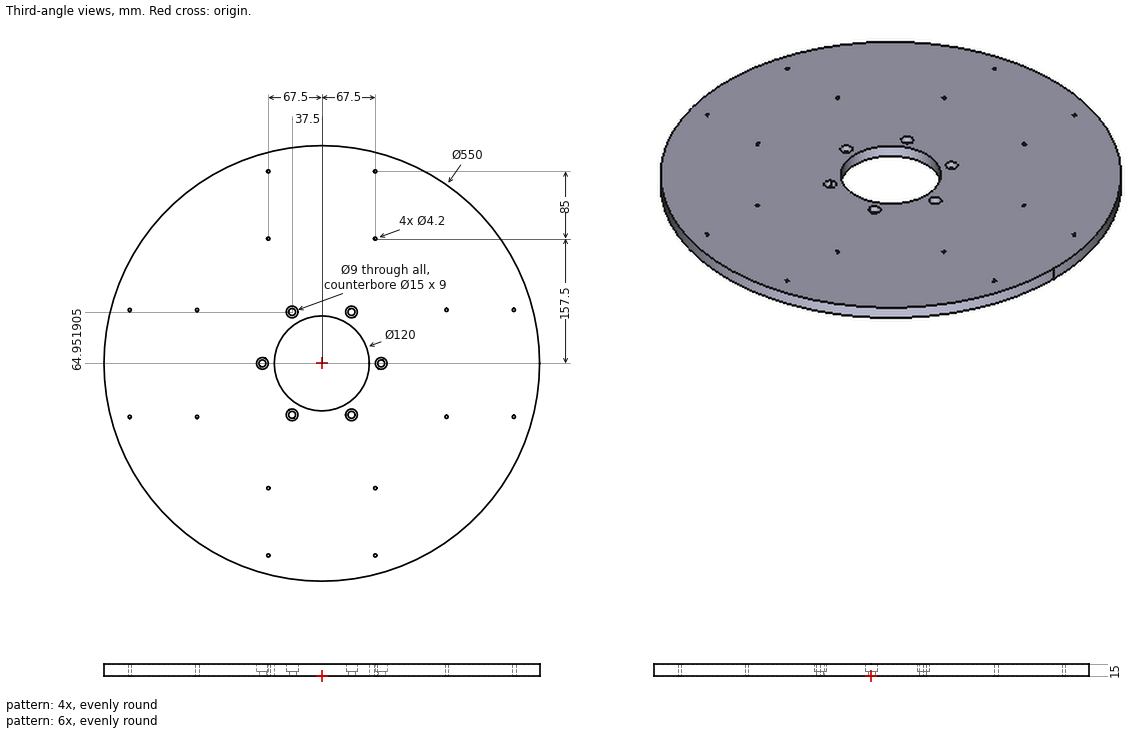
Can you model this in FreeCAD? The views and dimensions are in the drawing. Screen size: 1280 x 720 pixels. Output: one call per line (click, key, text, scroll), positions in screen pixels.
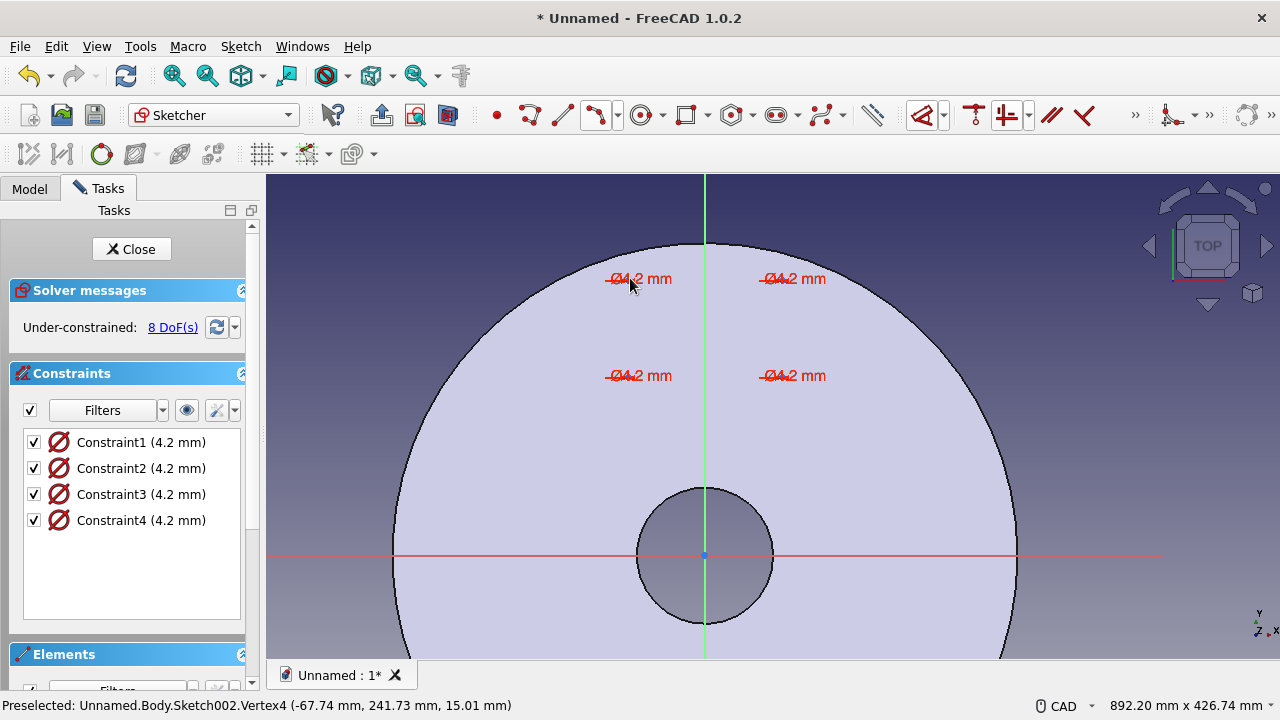
click(782, 378)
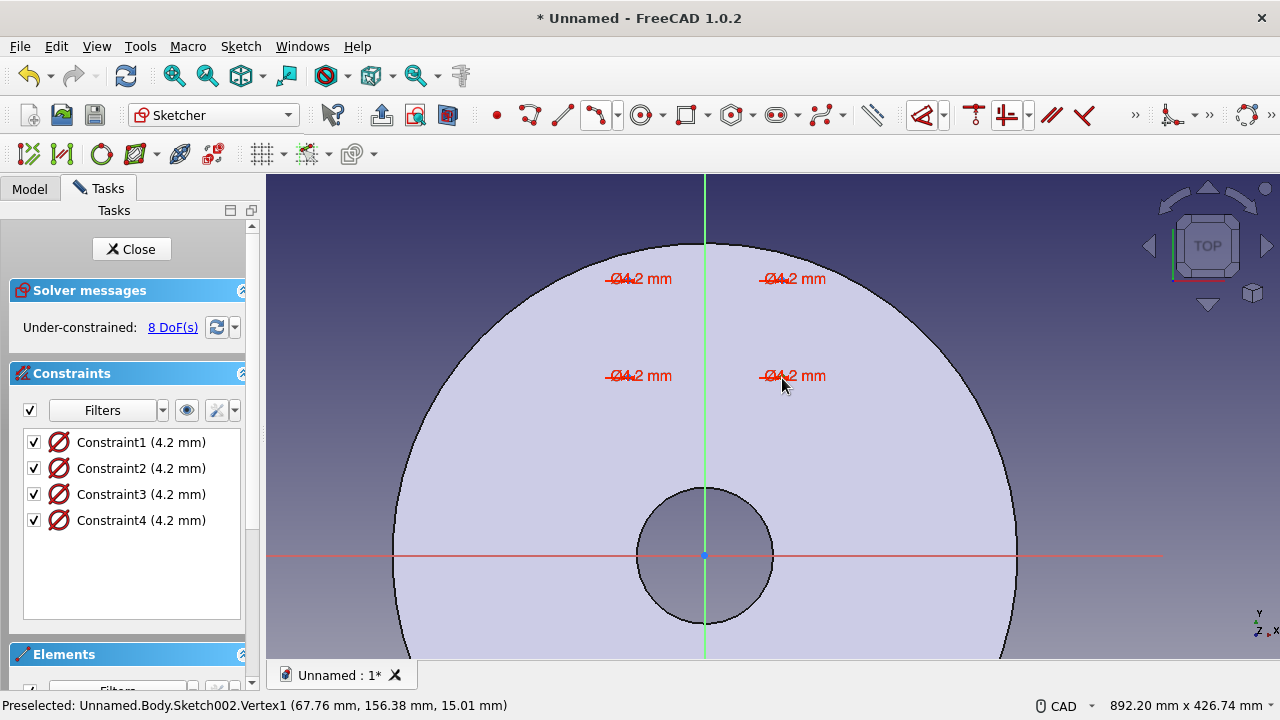
click(782, 281)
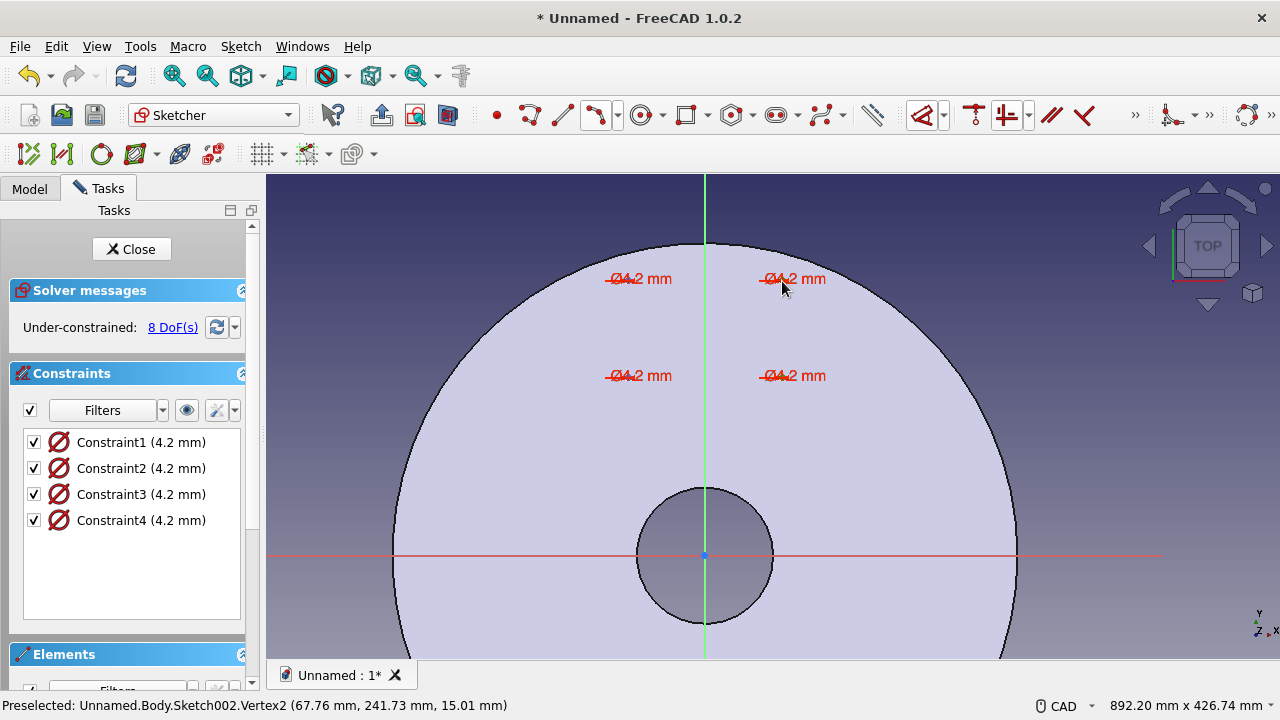
click(1028, 116)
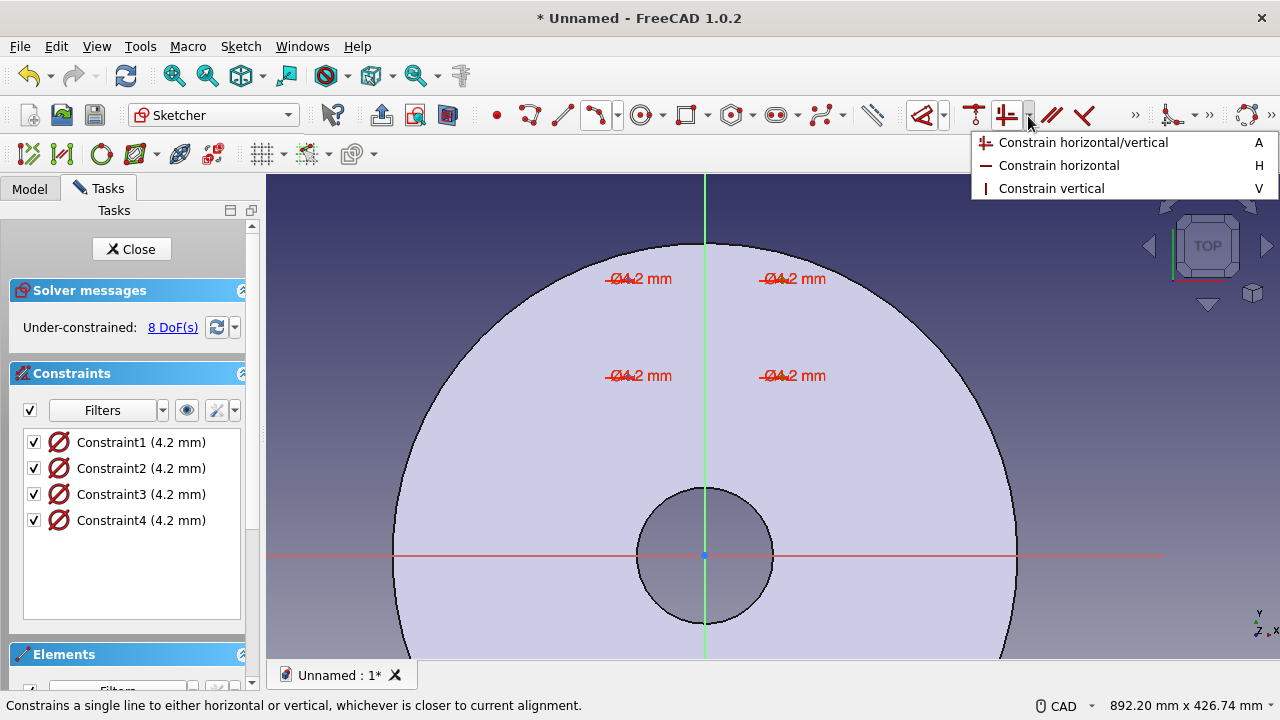
click(1125, 188)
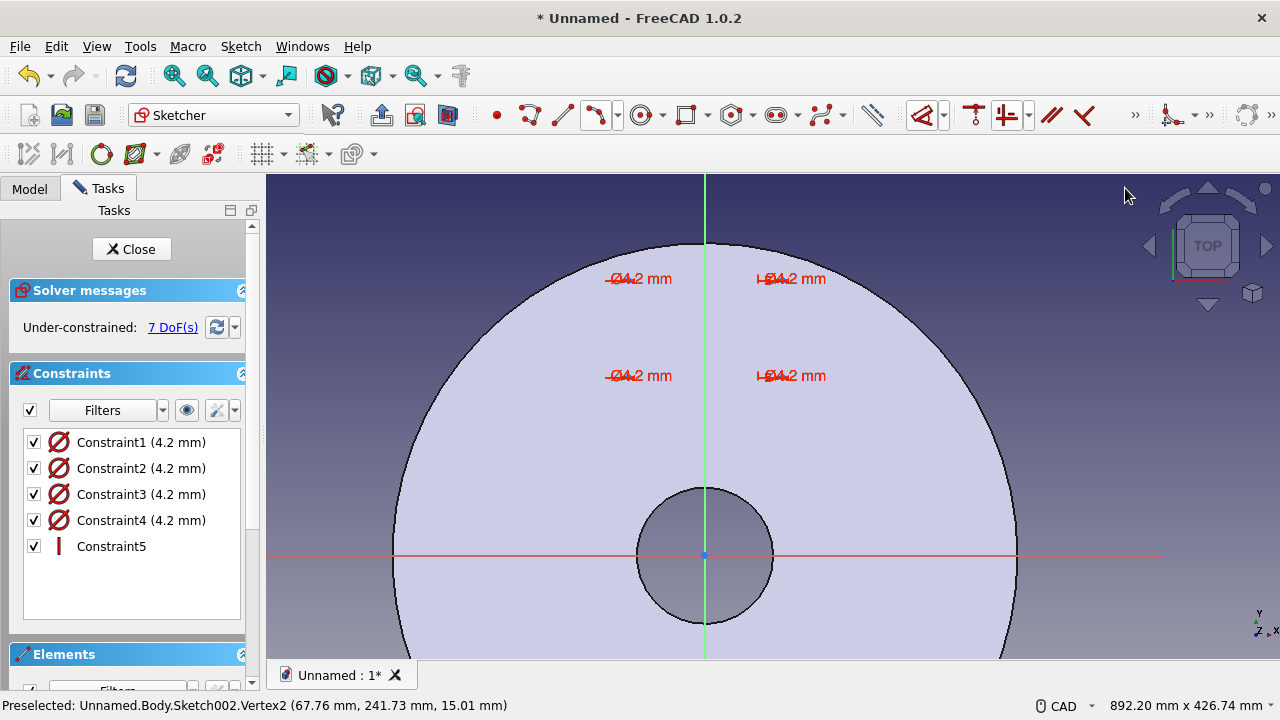
click(782, 378)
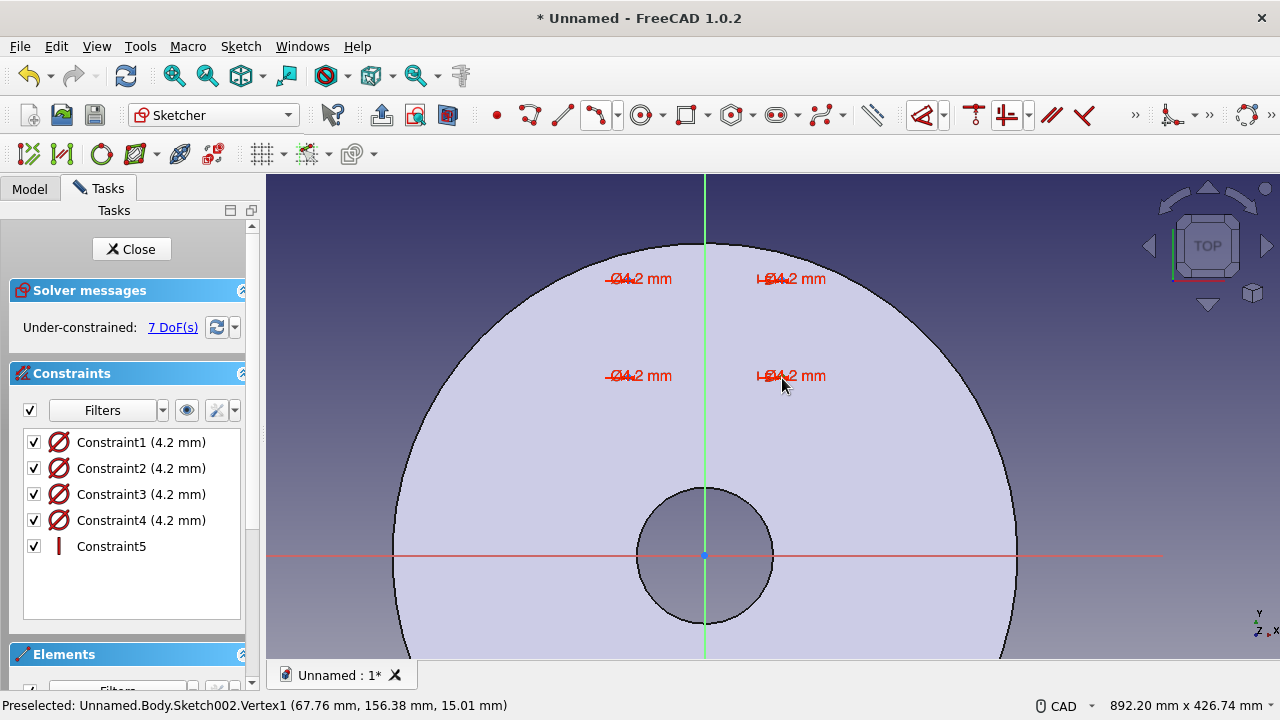
click(628, 378)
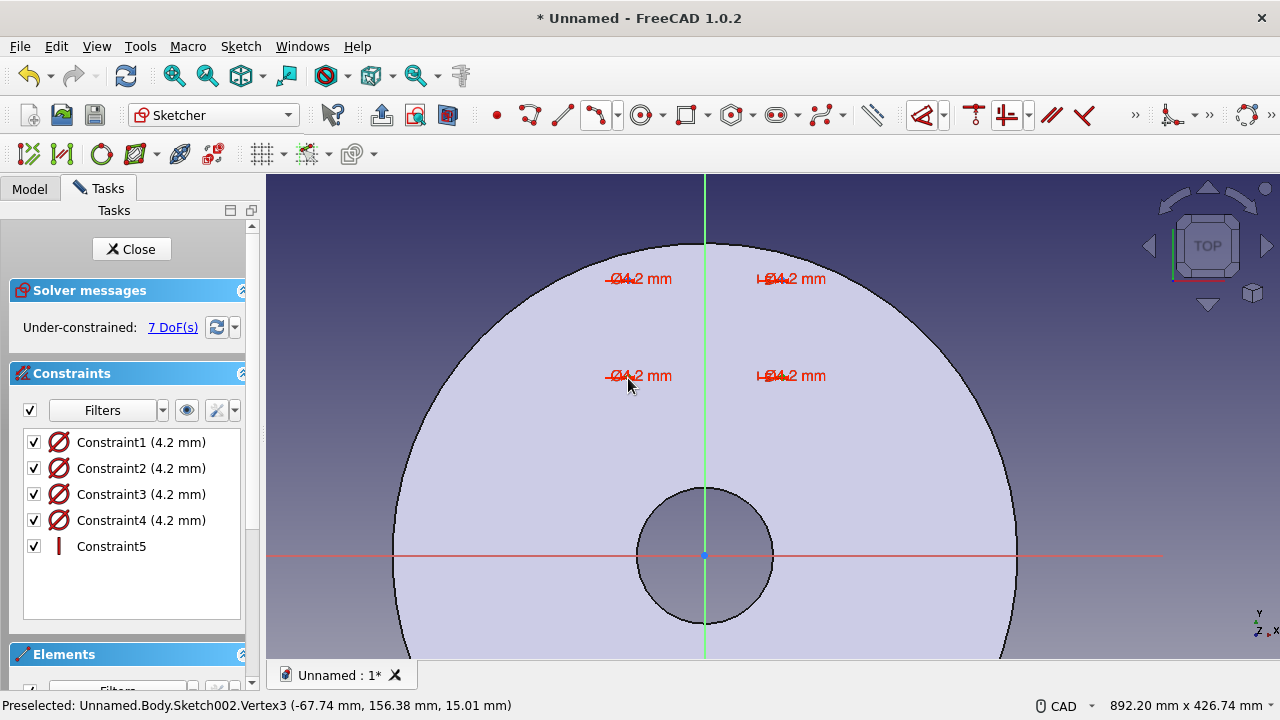
key(h)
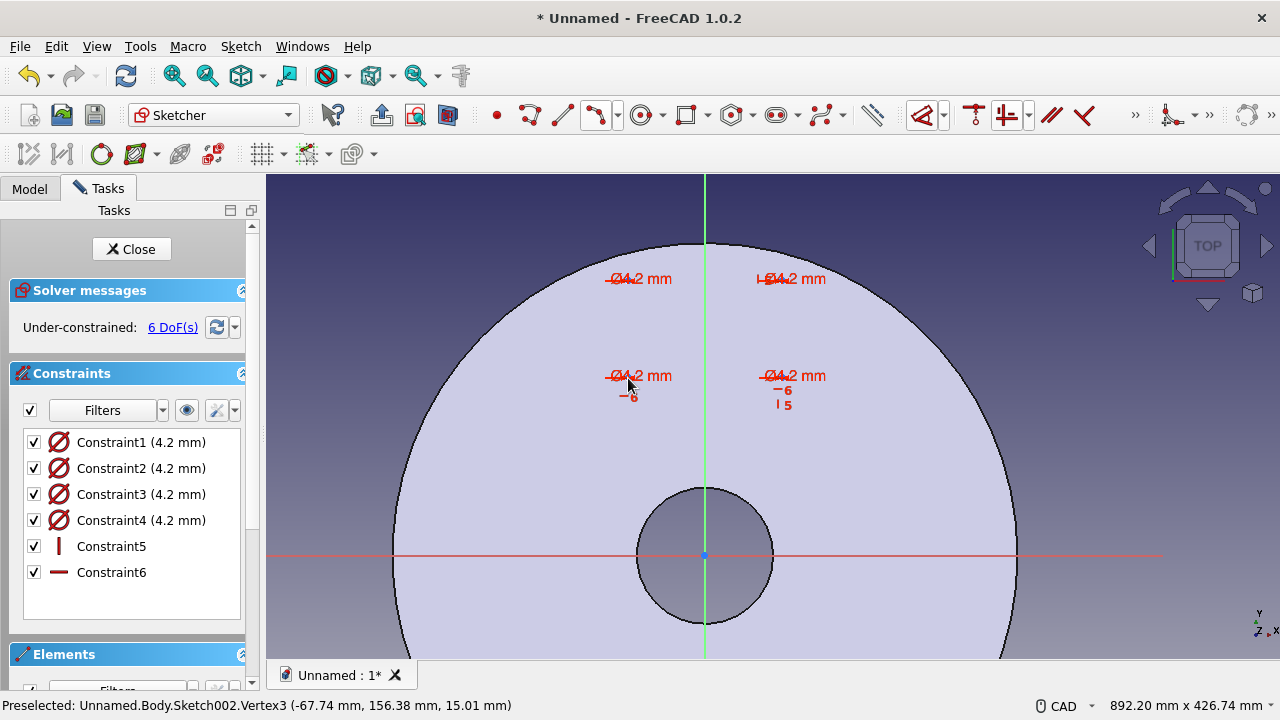
click(628, 378)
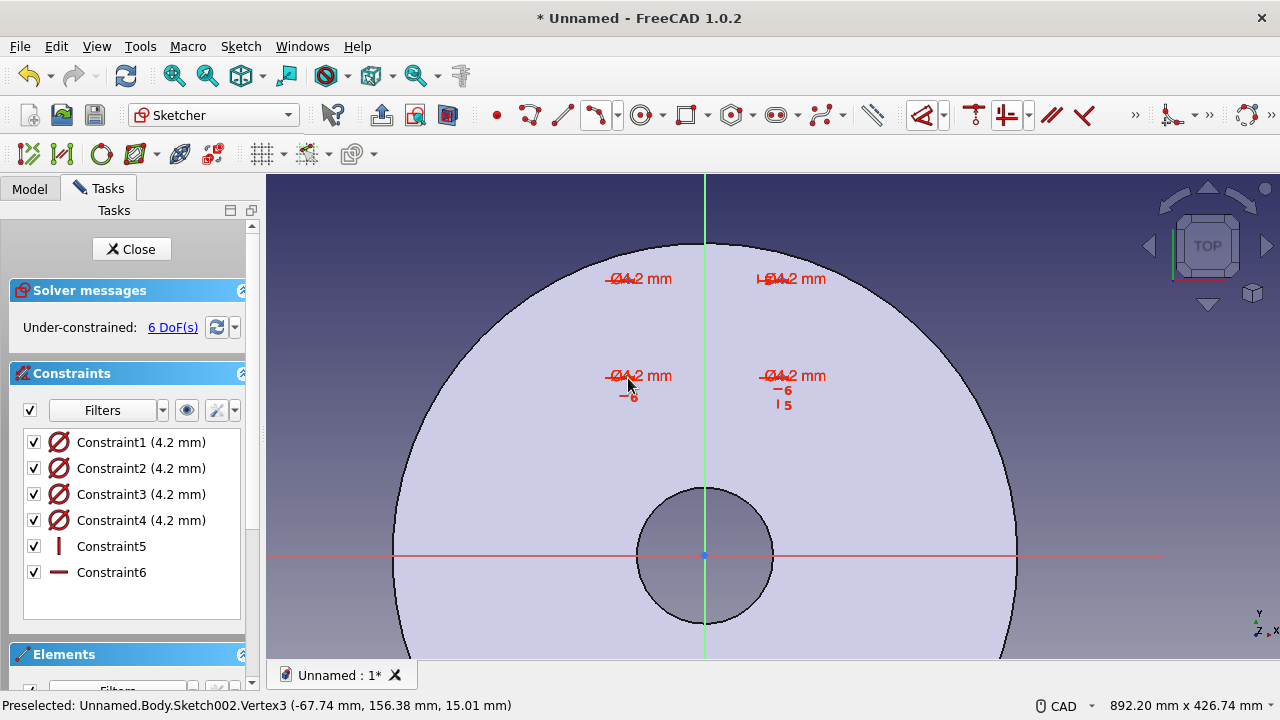
click(628, 281)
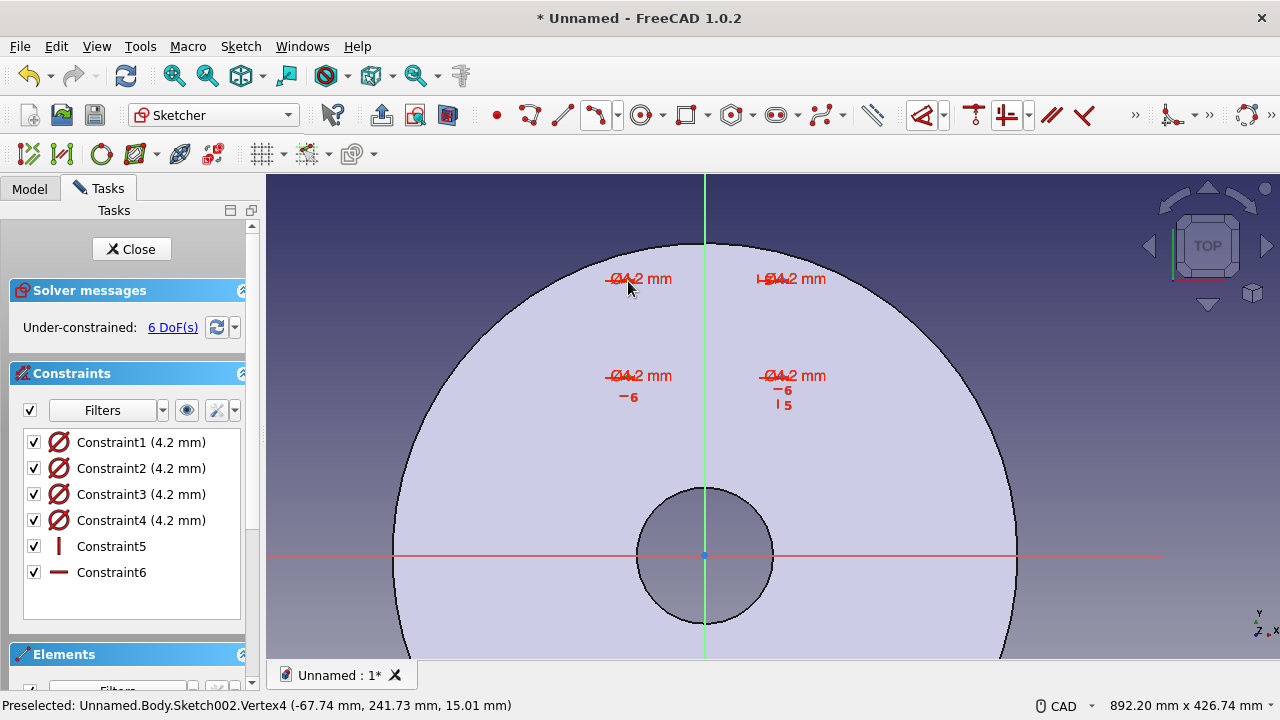
click(1028, 116)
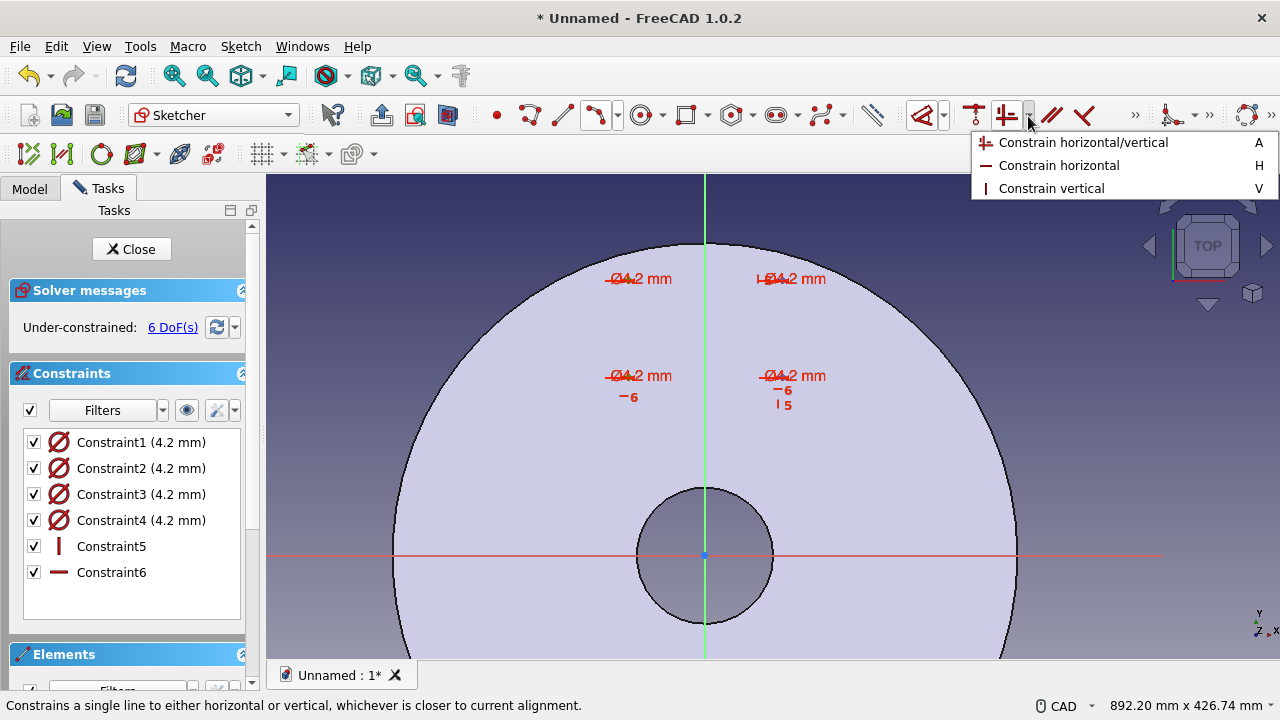
click(1125, 188)